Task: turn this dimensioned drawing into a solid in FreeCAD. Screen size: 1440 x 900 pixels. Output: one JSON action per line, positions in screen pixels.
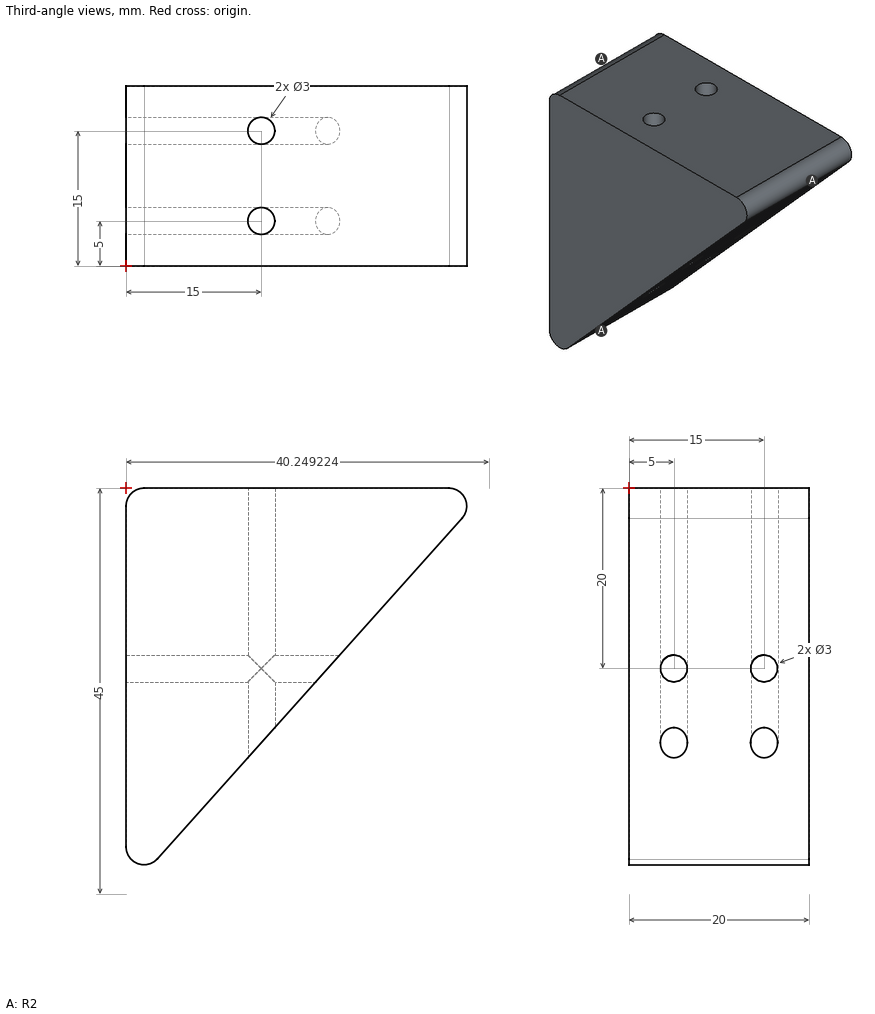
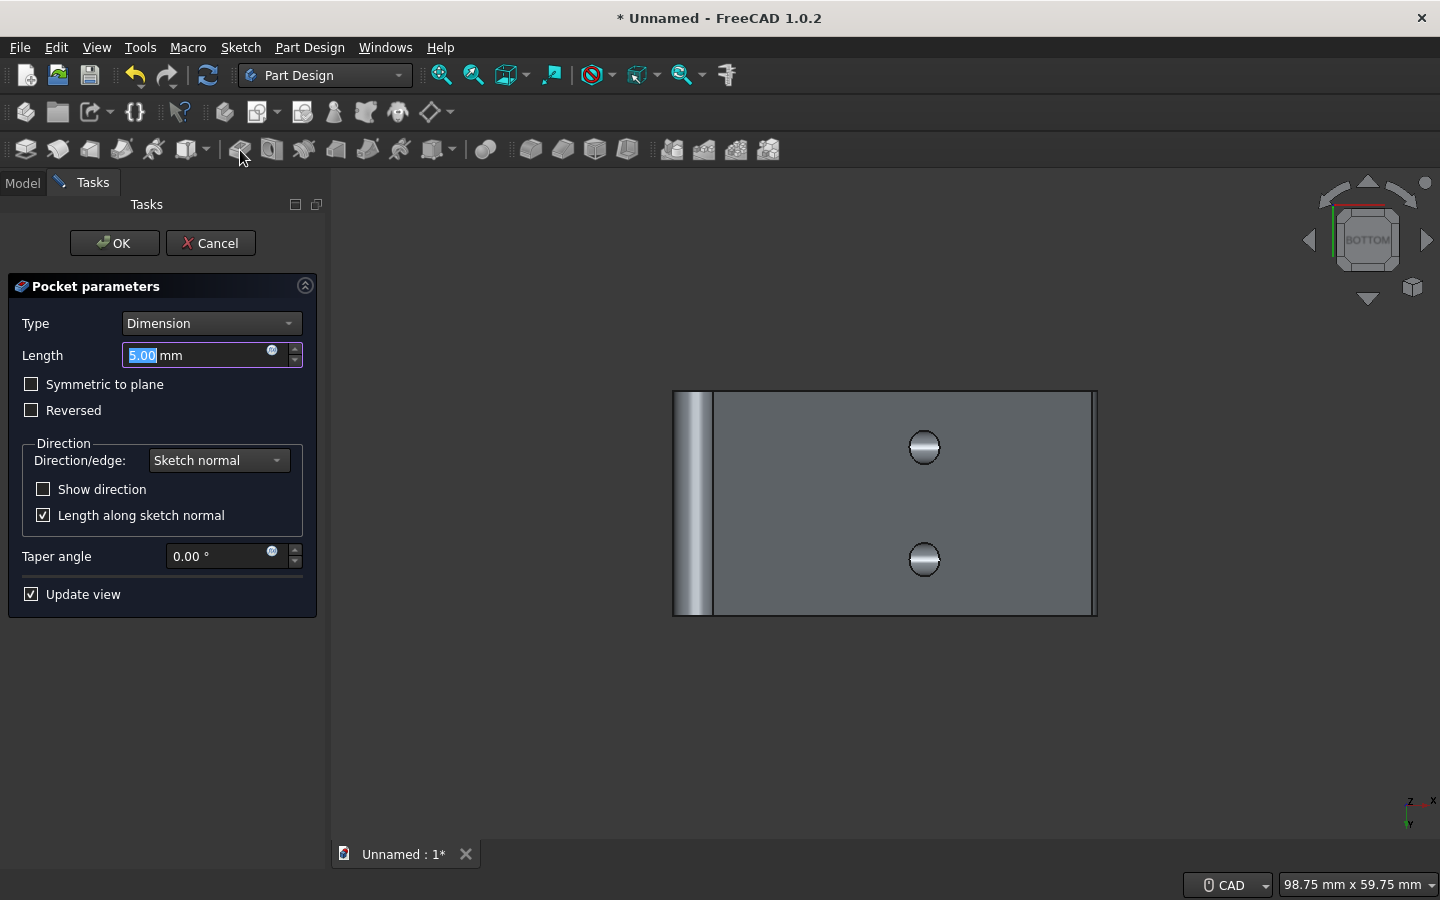
{"action": "left_click", "coordinate": [212, 324]}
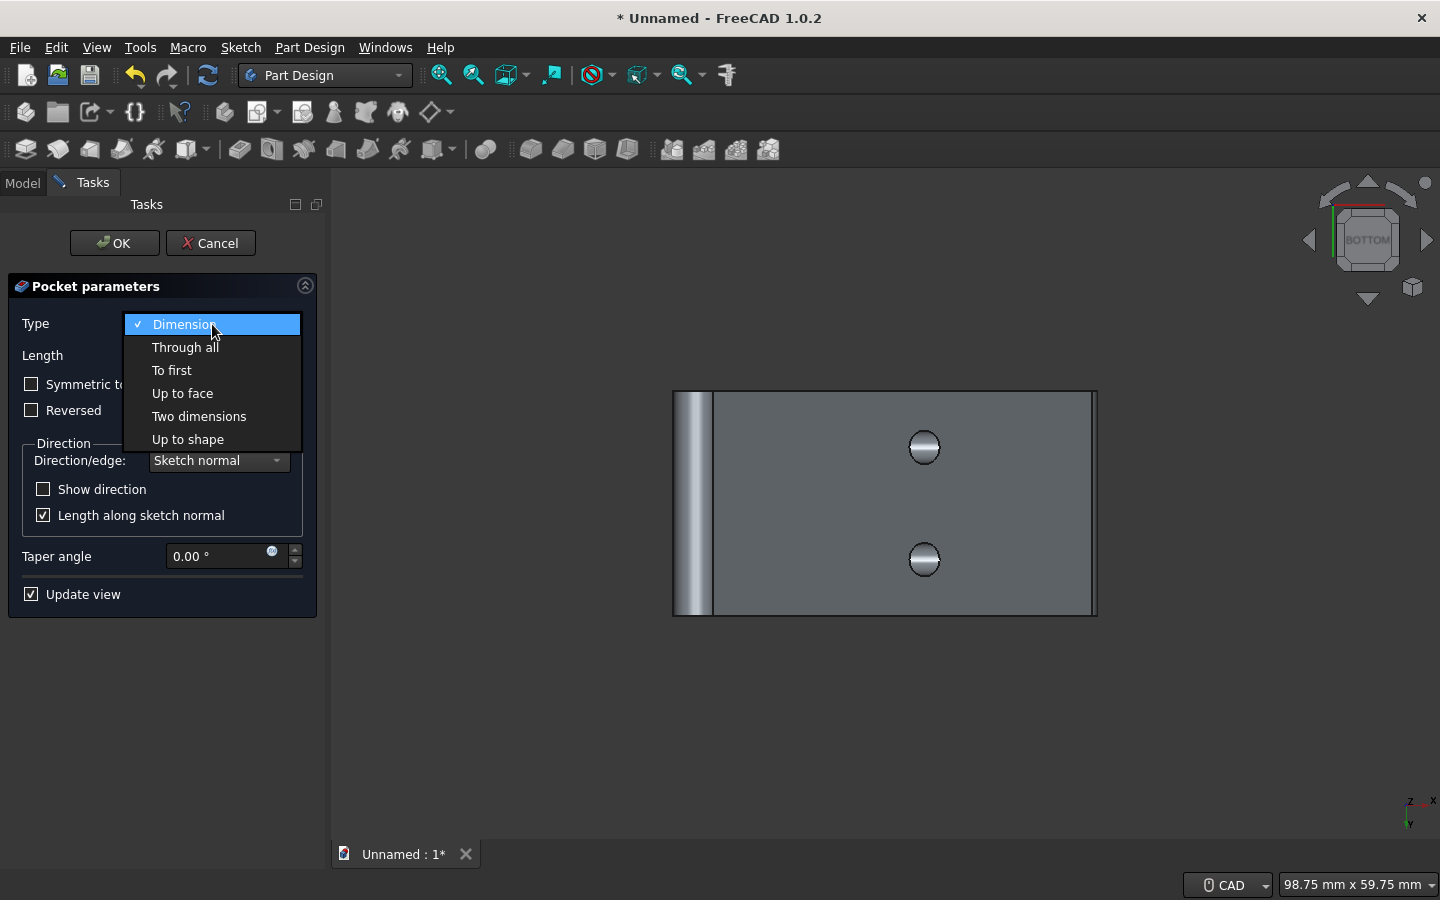
{"action": "left_click", "coordinate": [212, 348]}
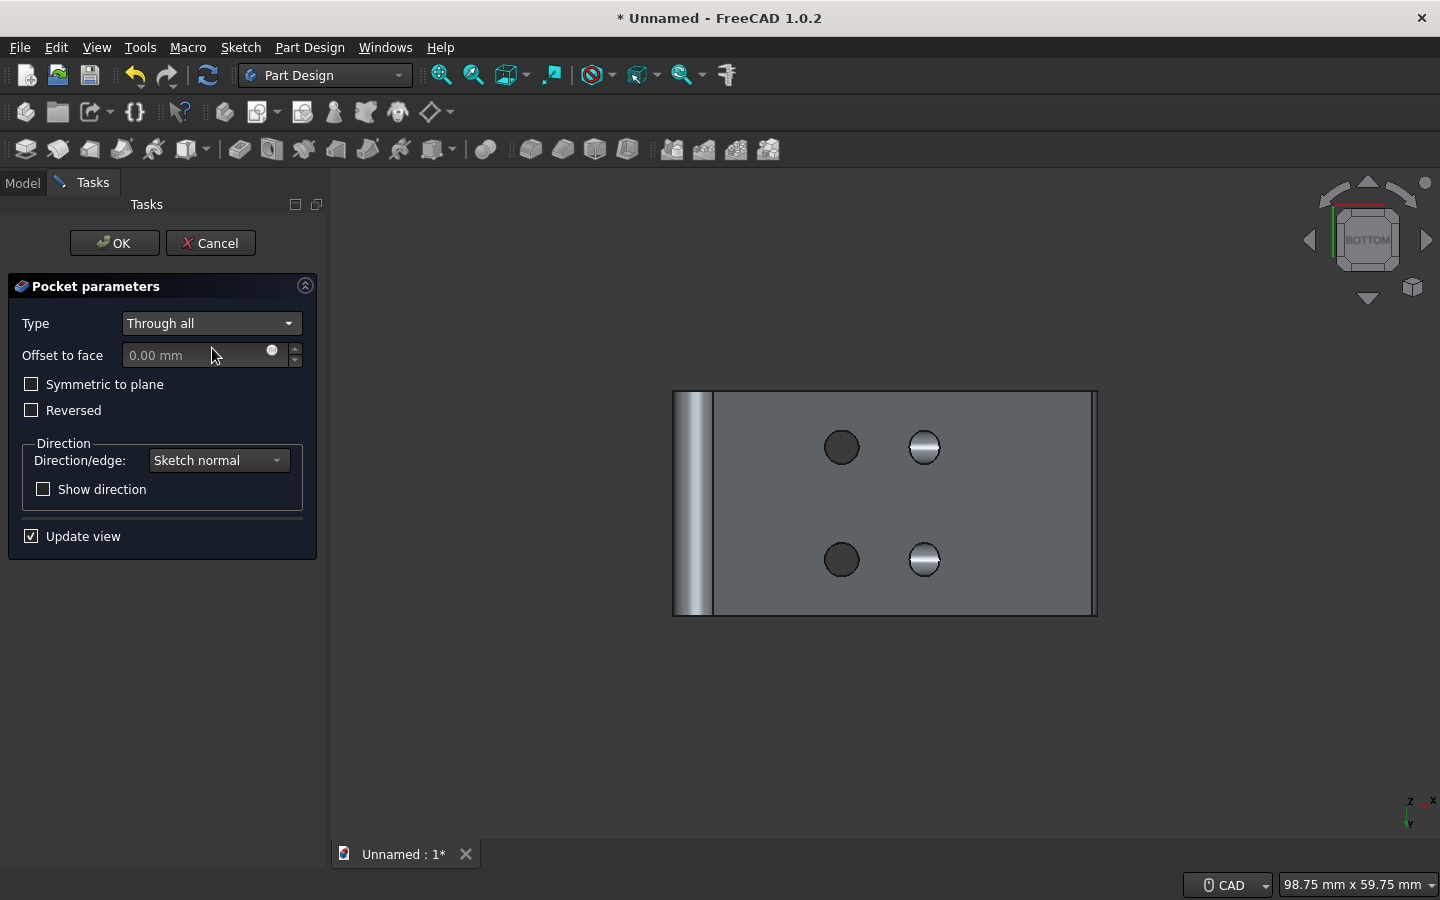
{"action": "left_click", "coordinate": [115, 243]}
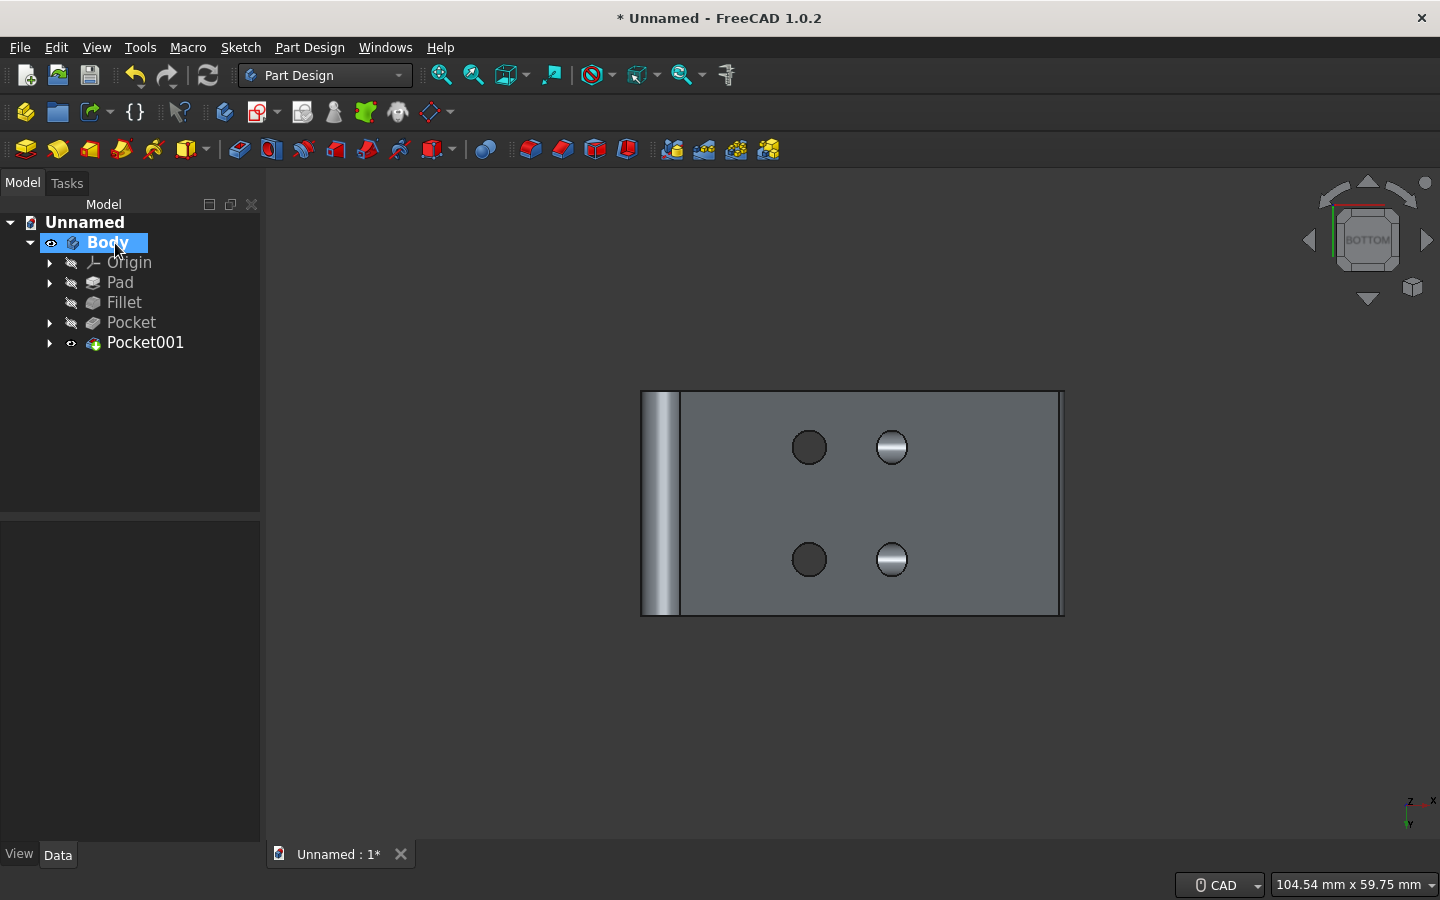
{"action": "key", "text": "0"}